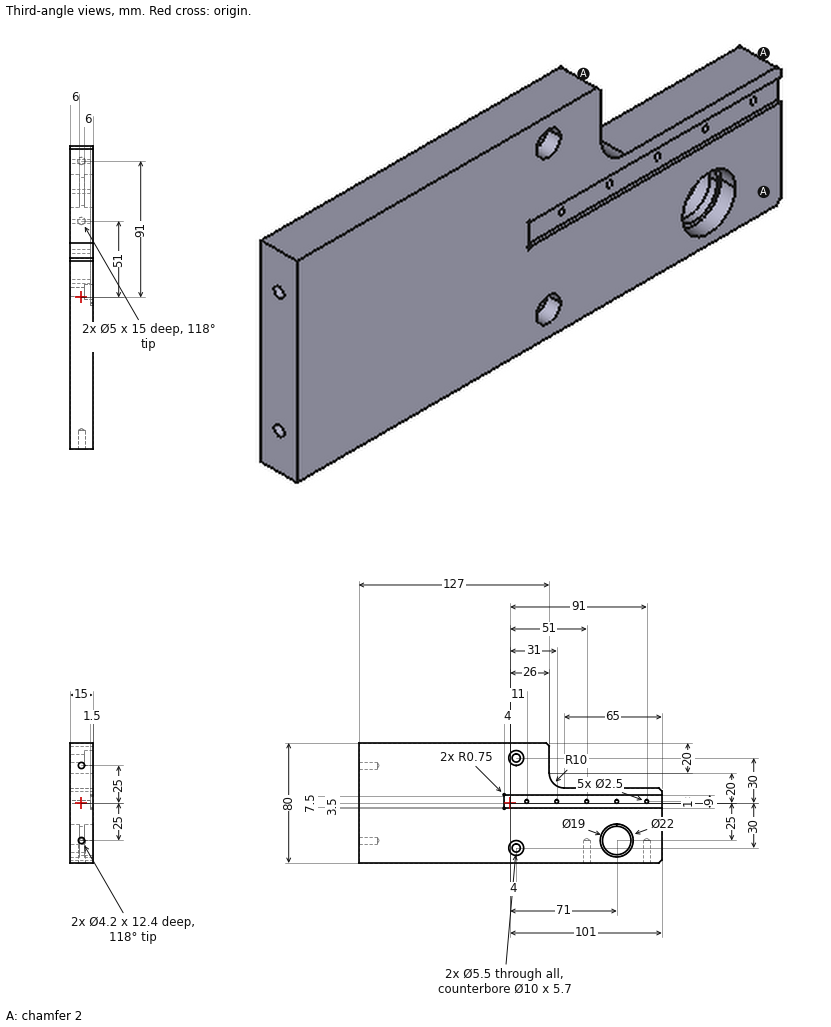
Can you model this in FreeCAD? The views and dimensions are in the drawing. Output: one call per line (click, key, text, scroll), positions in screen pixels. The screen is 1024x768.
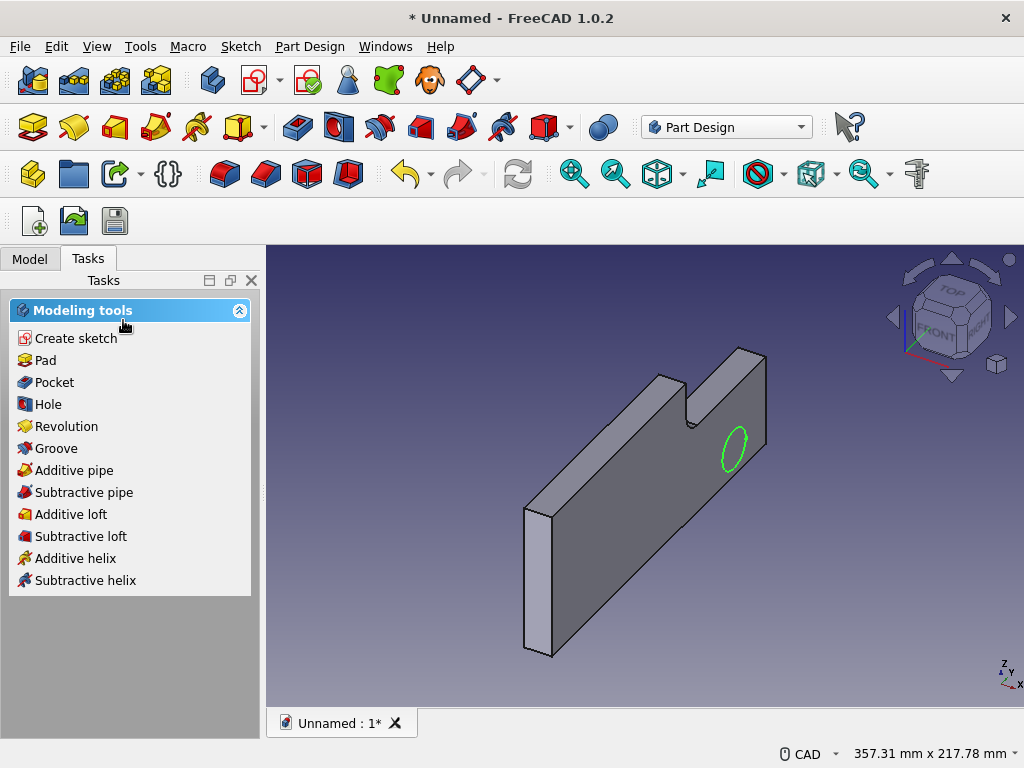
click(298, 128)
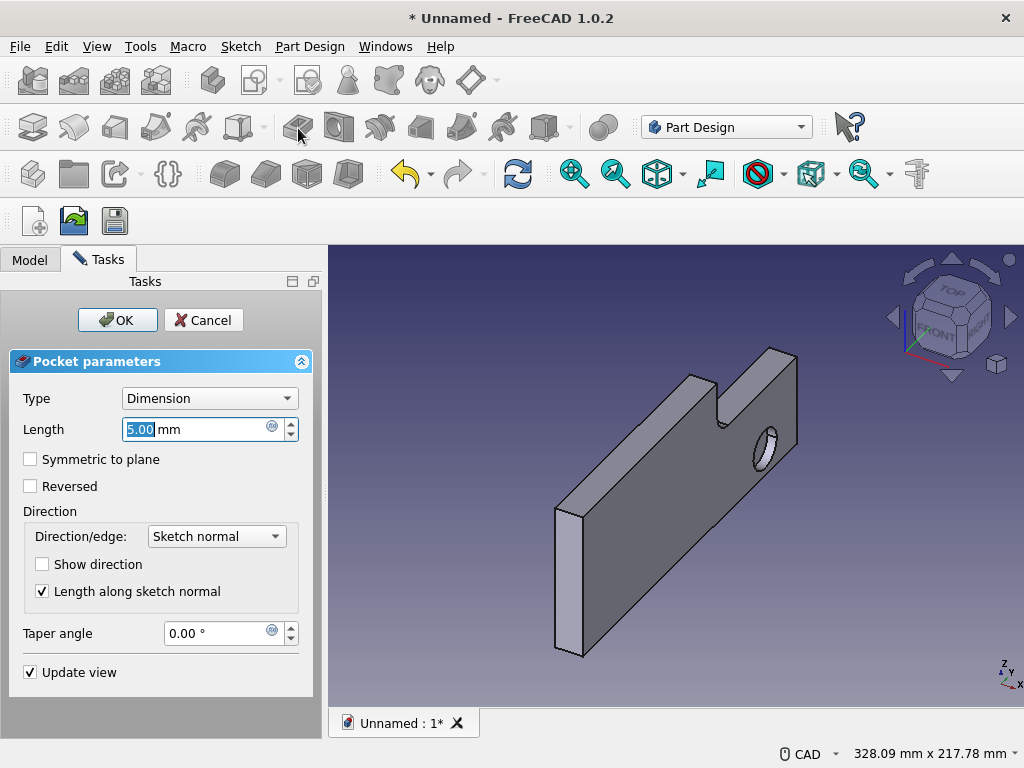
text(6)
key(Tab)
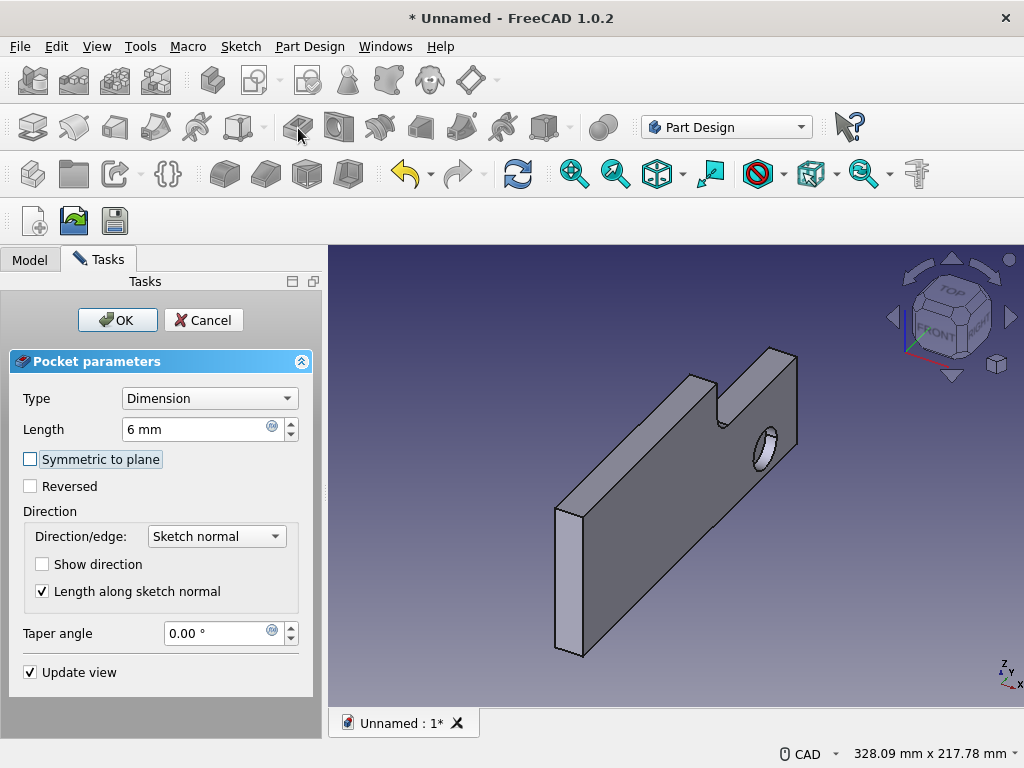
click(118, 320)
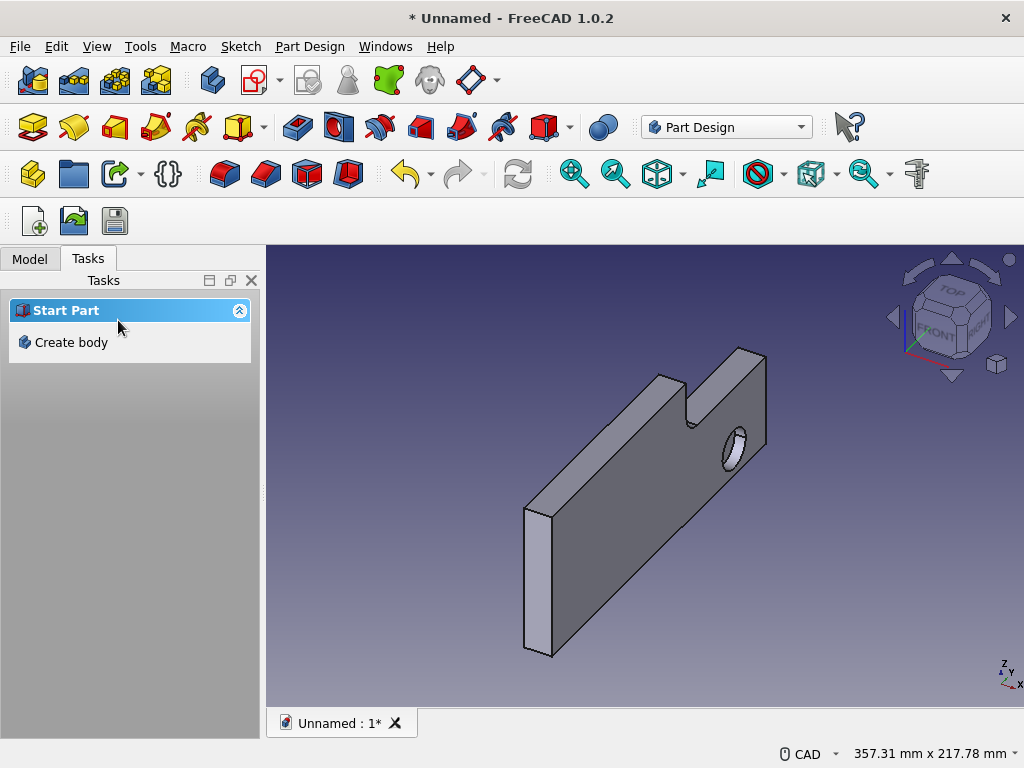
key(6)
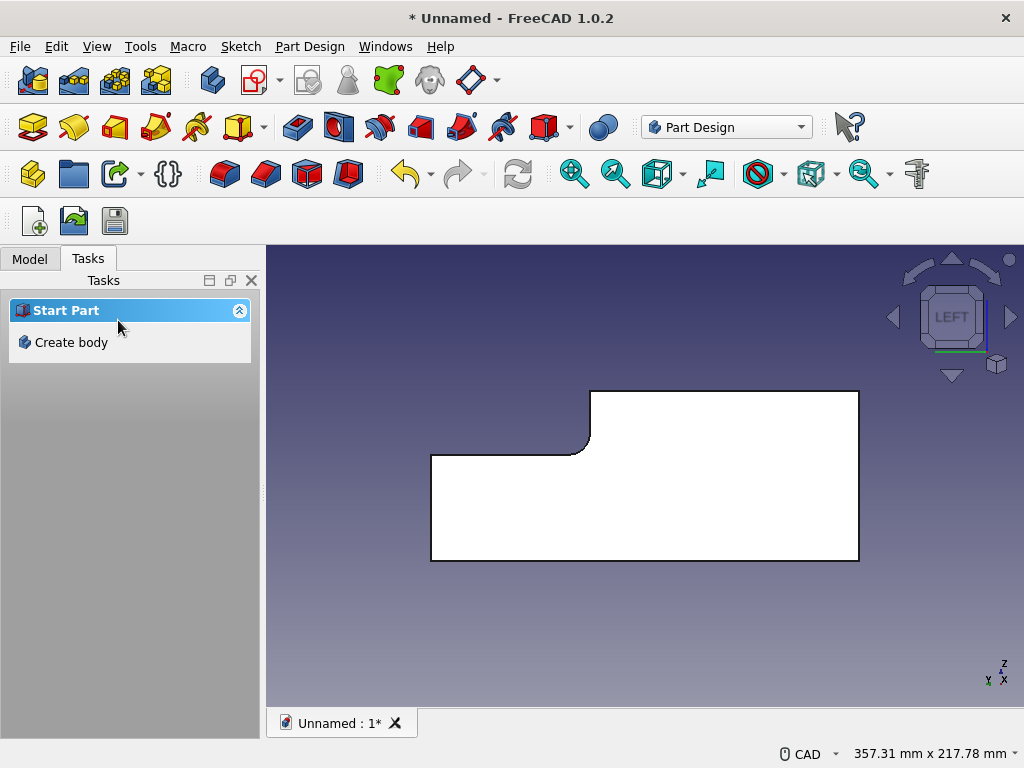
click(706, 475)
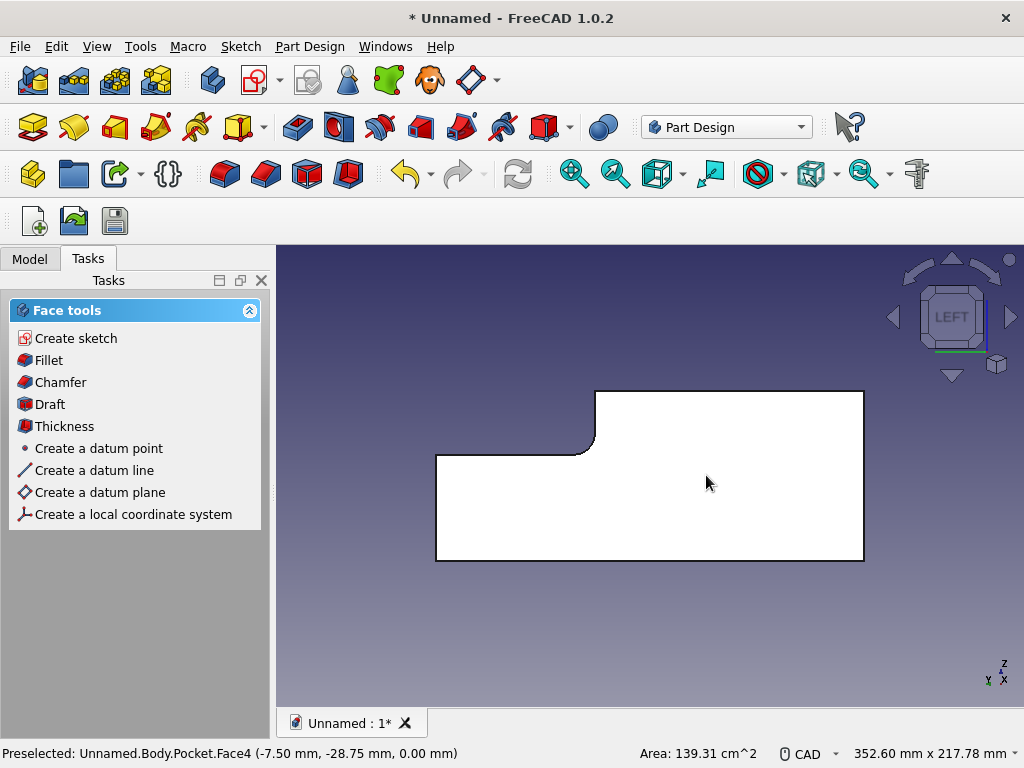
click(254, 80)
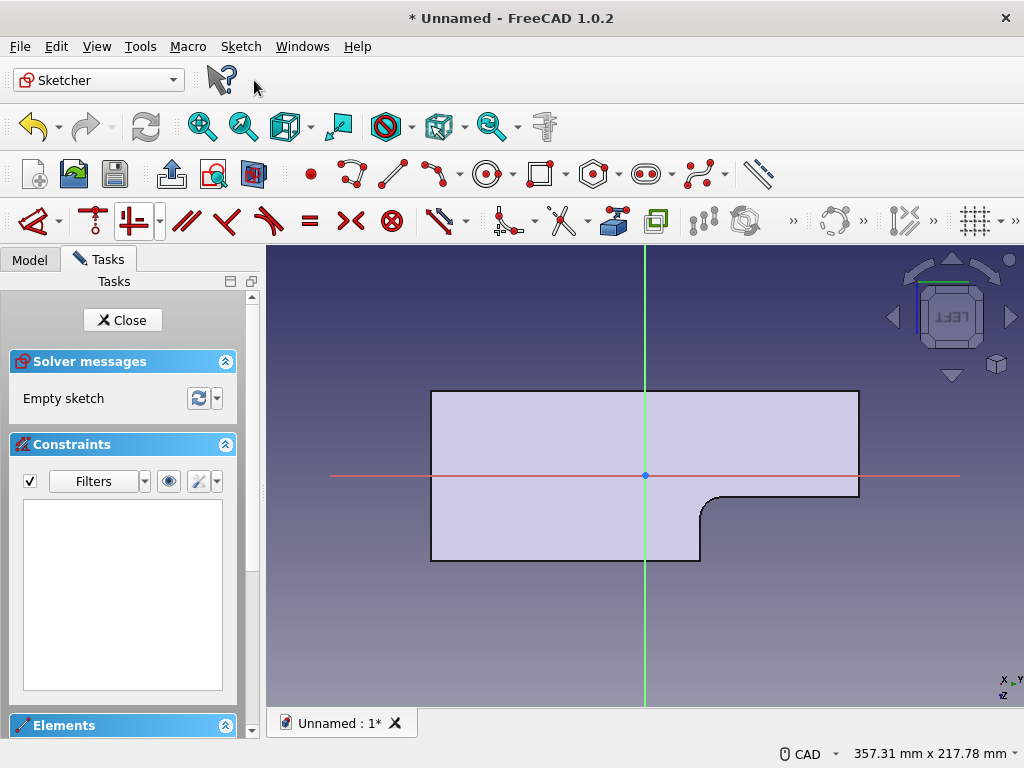
scroll(830, 415, up, 10)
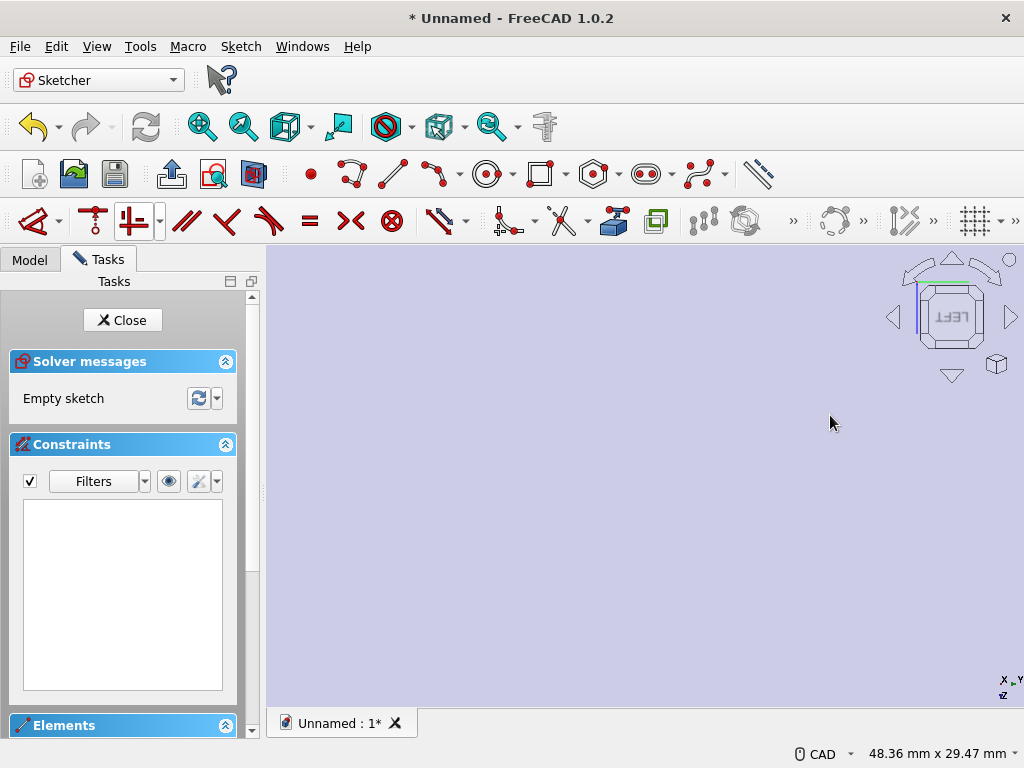
click(486, 174)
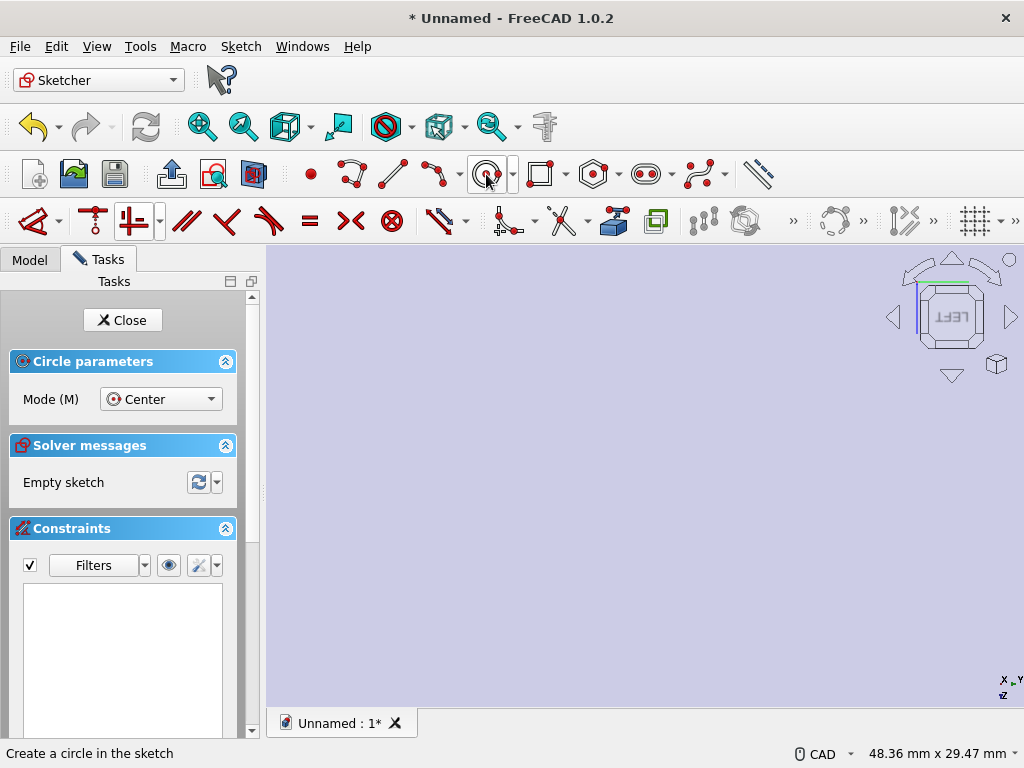
click(571, 472)
click(676, 366)
key(Escape)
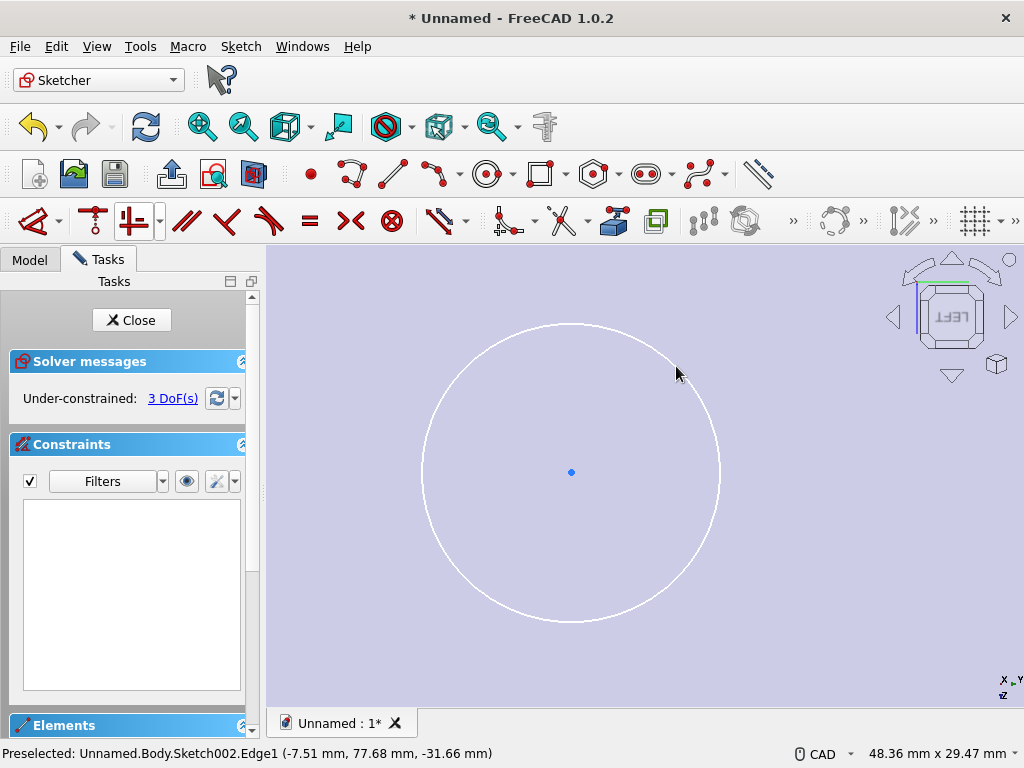
click(32, 222)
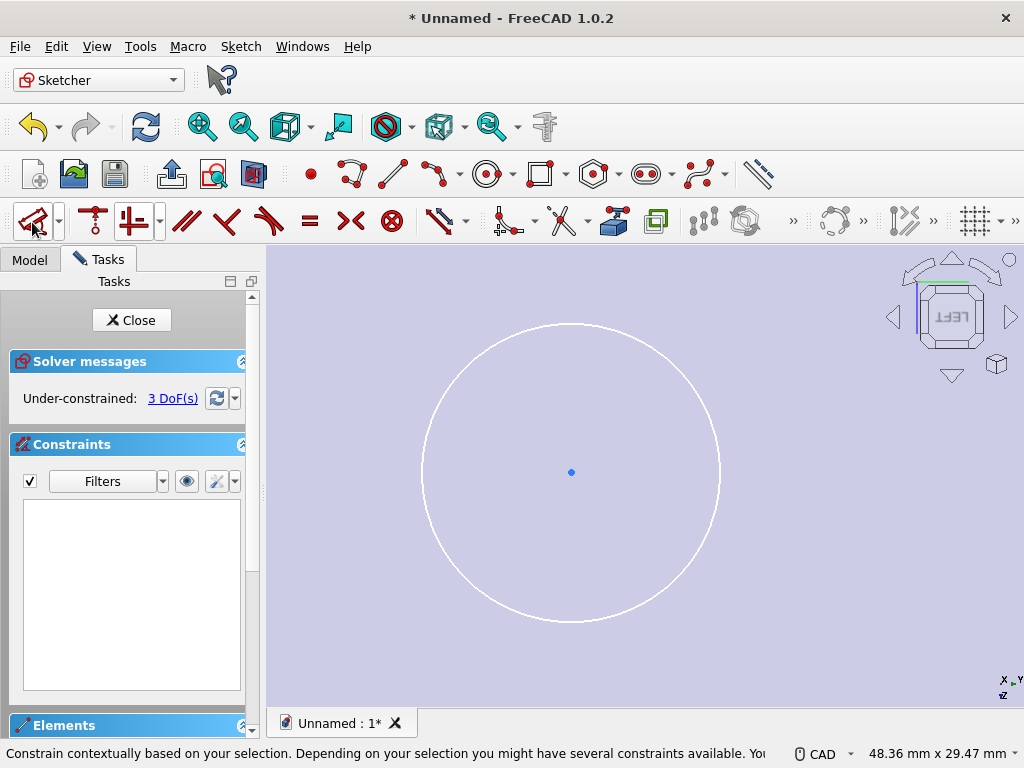
click(676, 367)
click(699, 344)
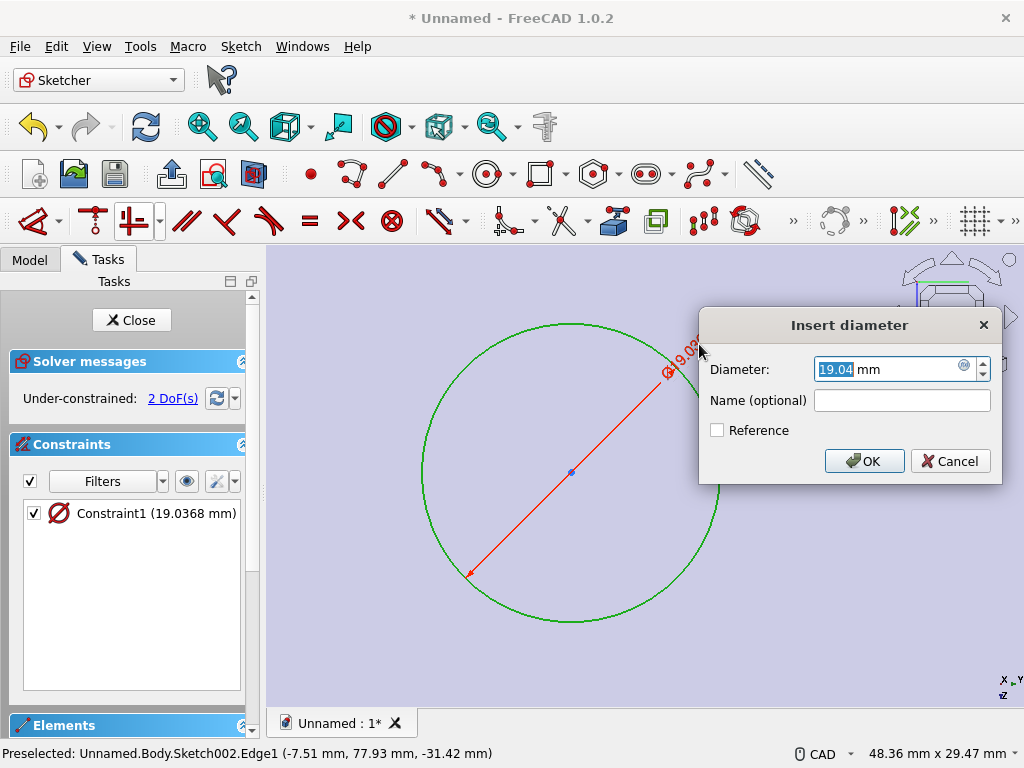
text(19)
key(Return)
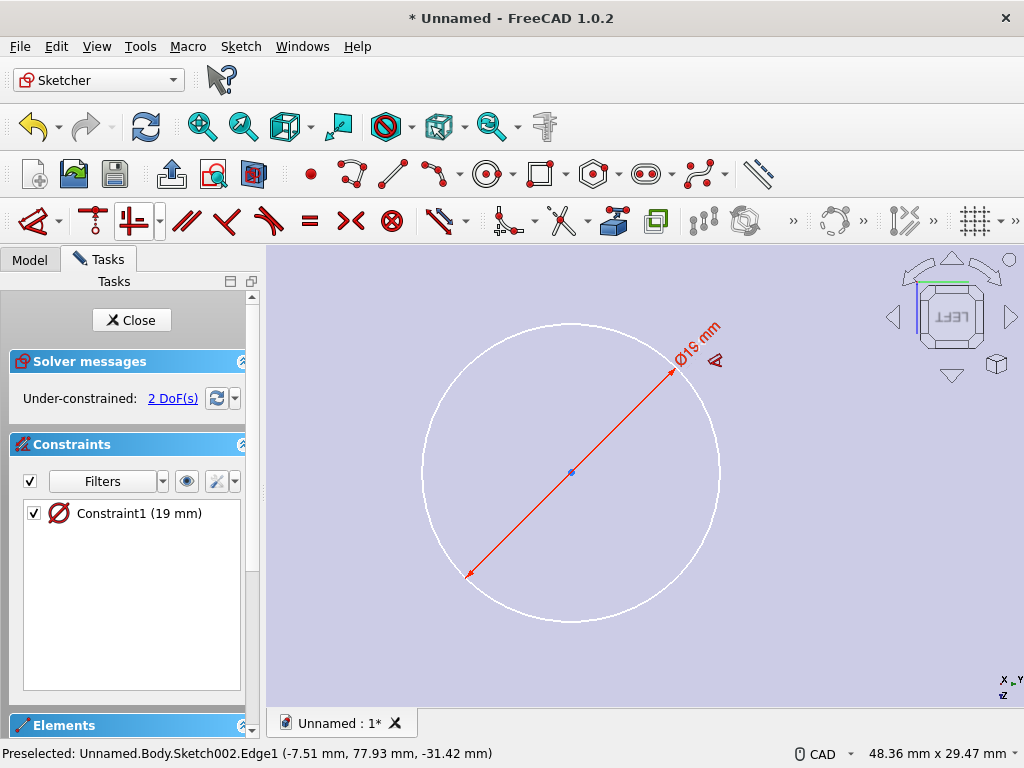
click(571, 473)
click(369, 439)